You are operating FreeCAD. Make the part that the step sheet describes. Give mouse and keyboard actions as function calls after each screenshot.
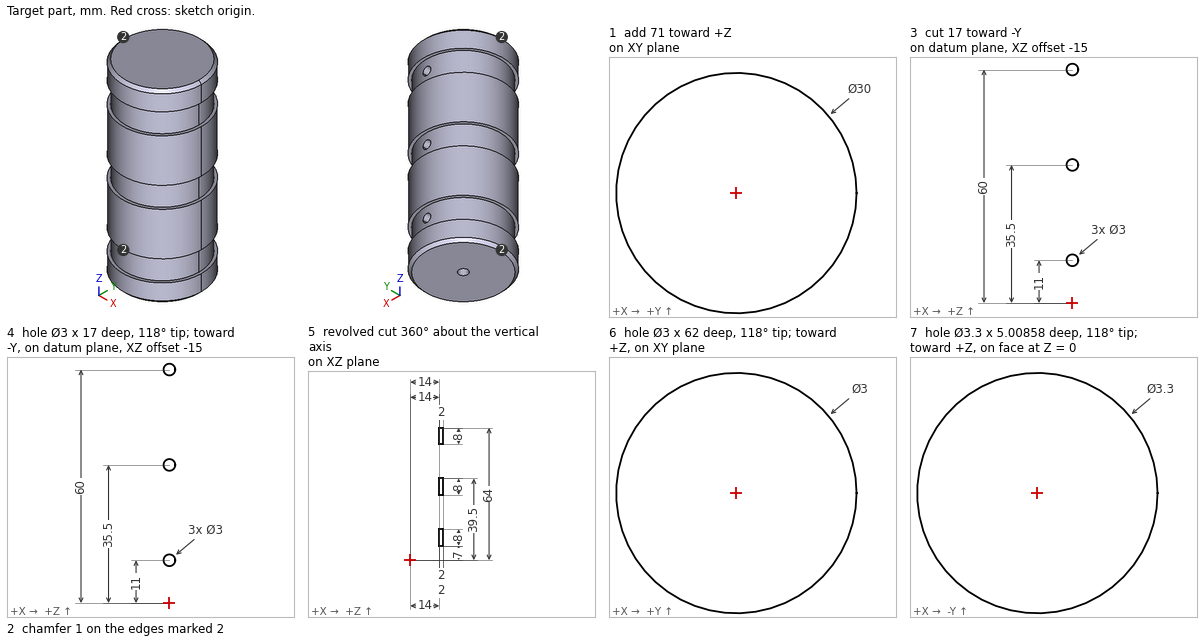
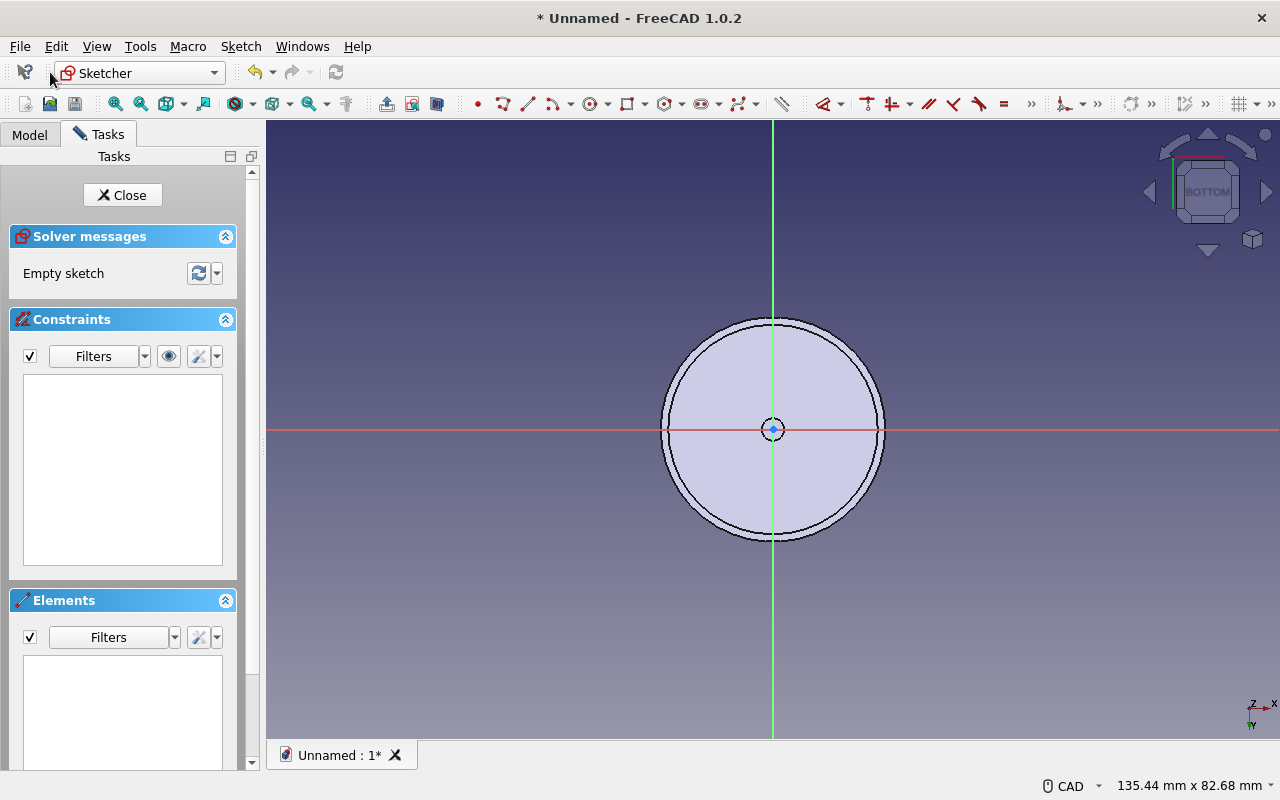
scroll(777, 430, up, 14)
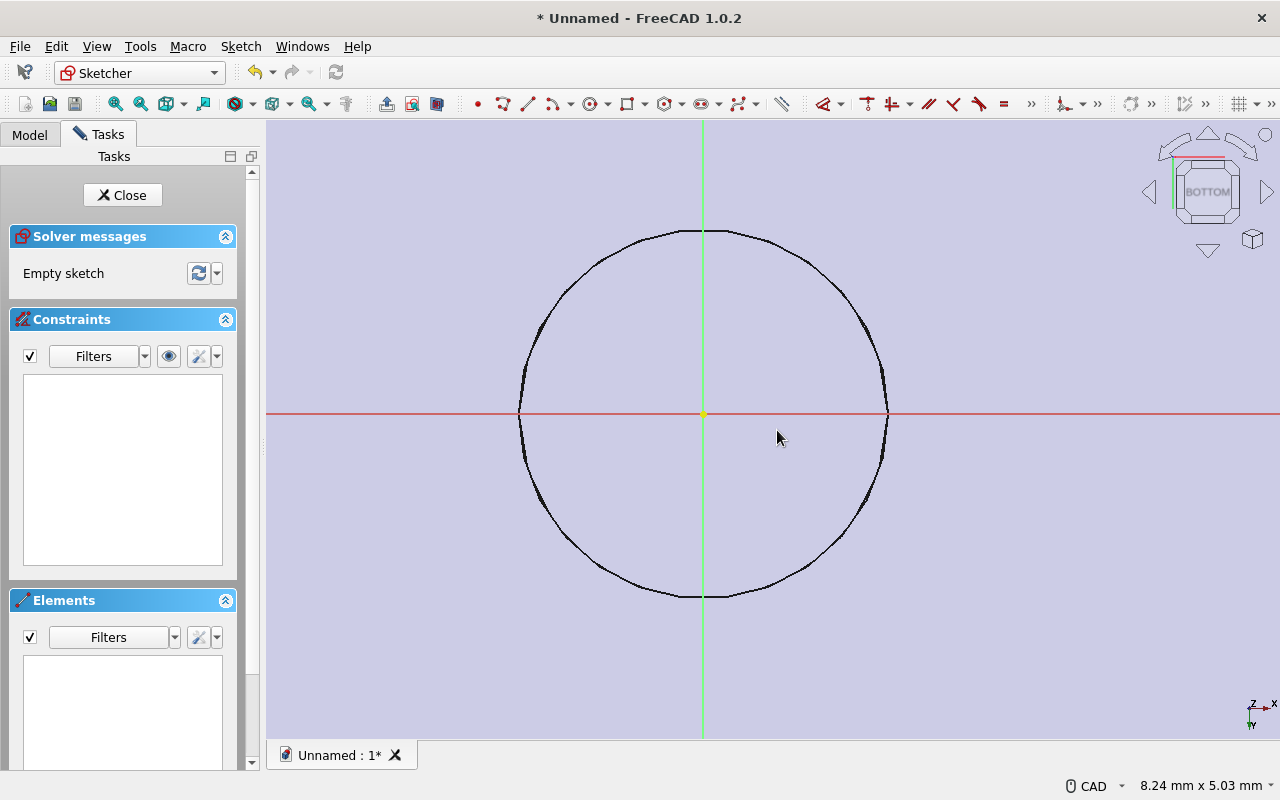
click(590, 104)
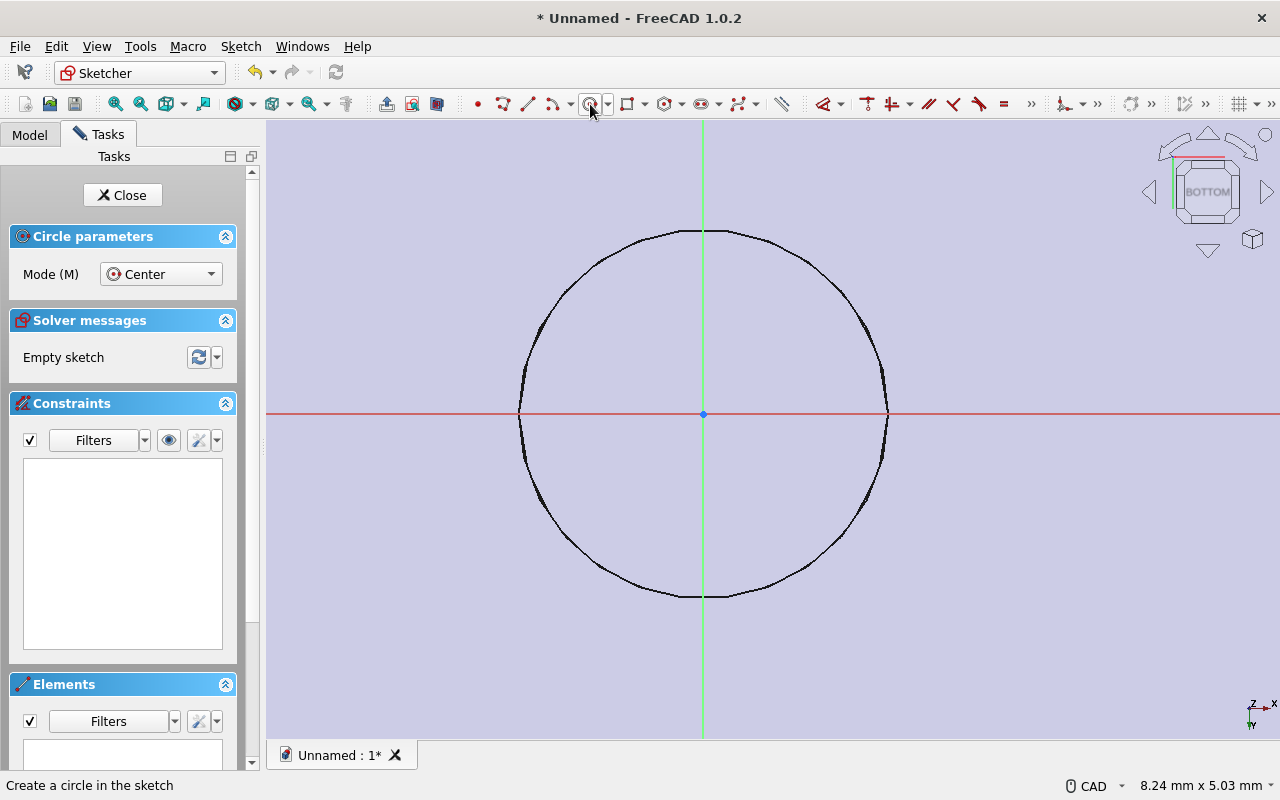
click(703, 414)
move(847, 270)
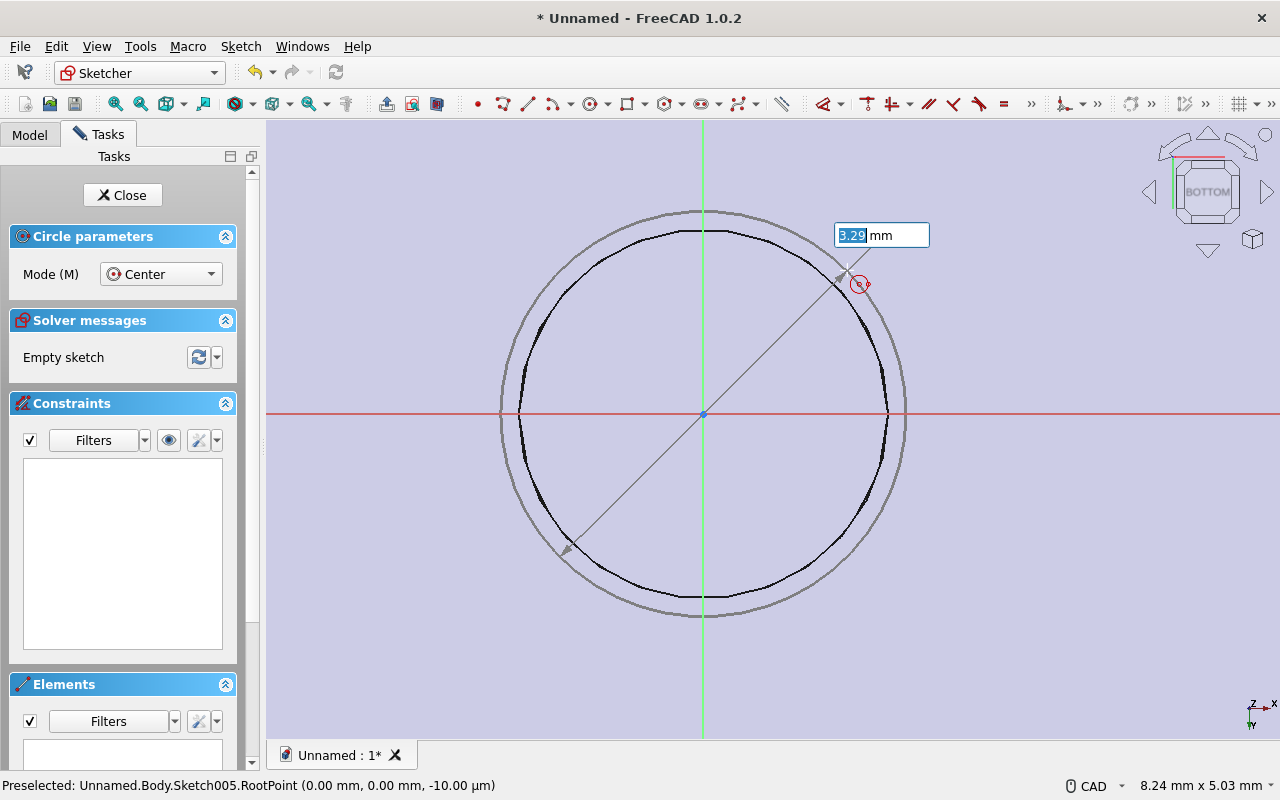
text(3.3)
key(Return)
key(Escape)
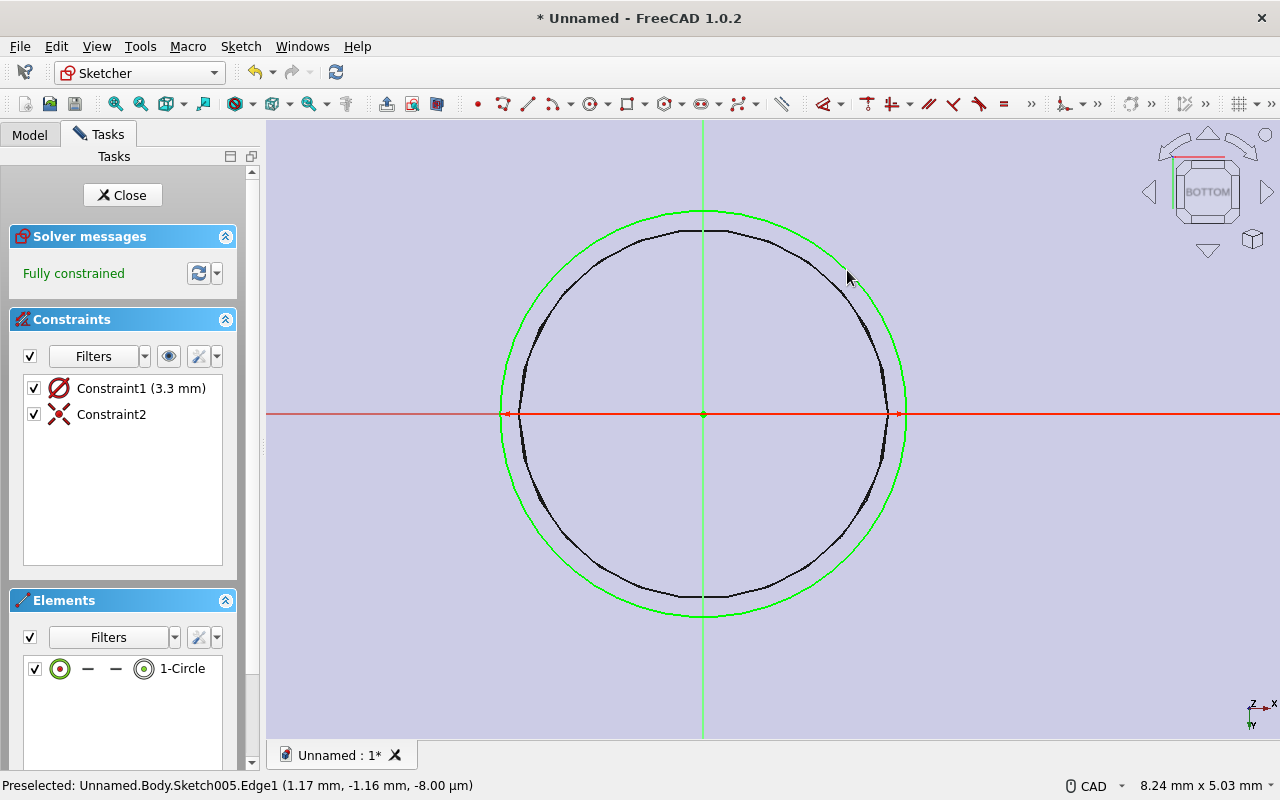
click(123, 195)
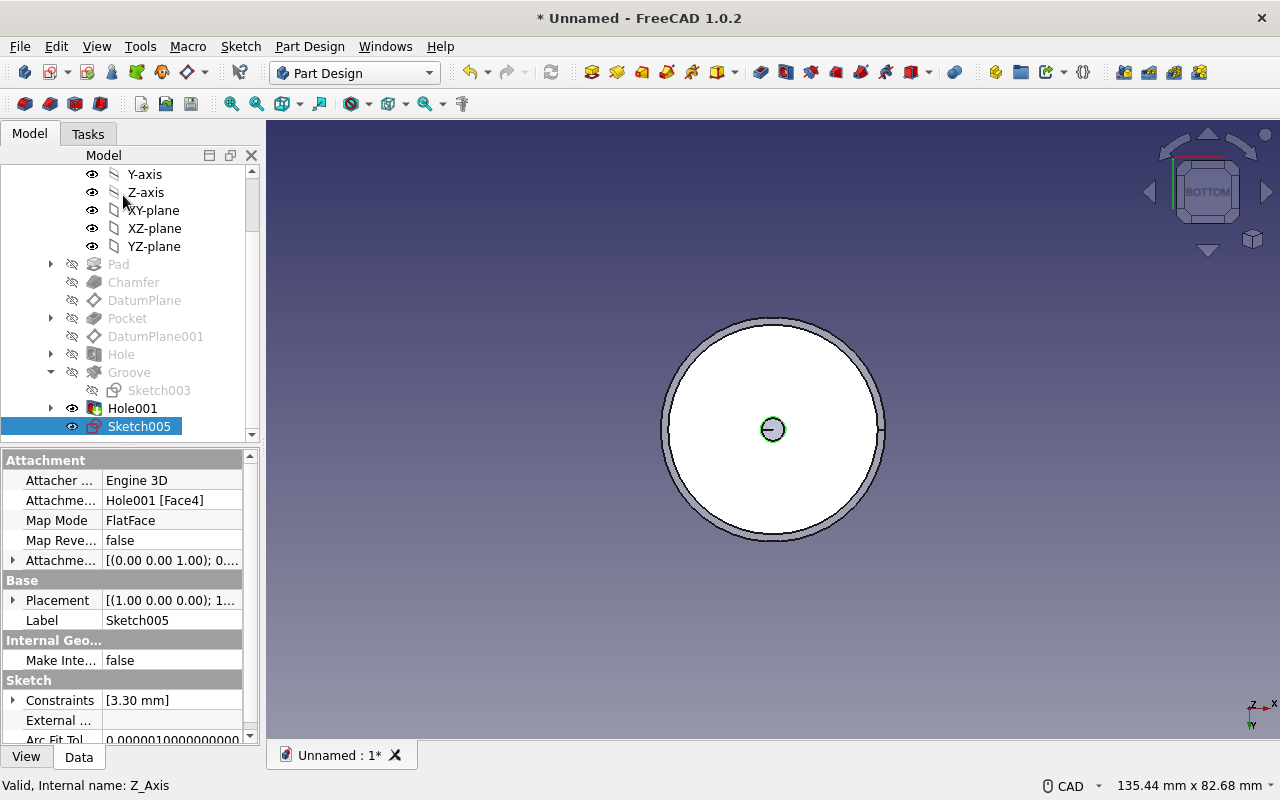
click(786, 72)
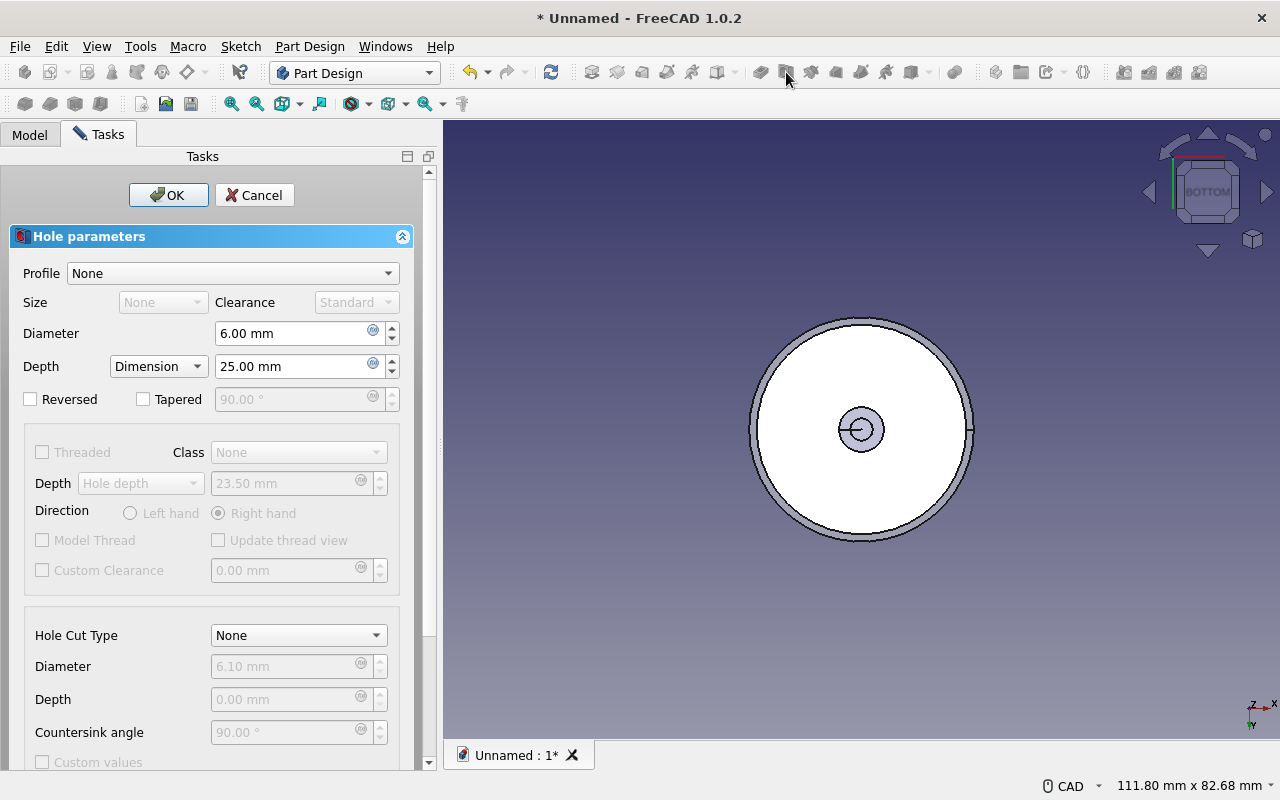
triple_click(300, 334)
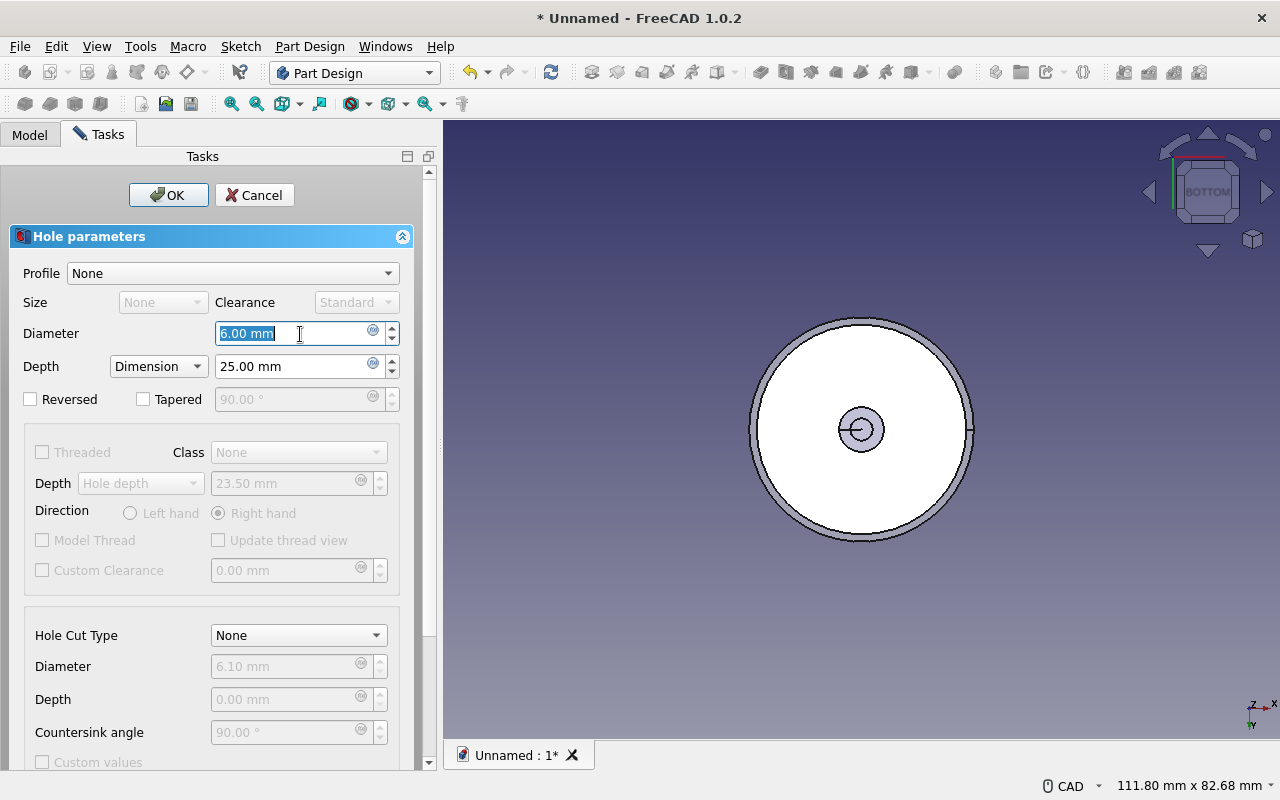
text(3.3)
key(Tab)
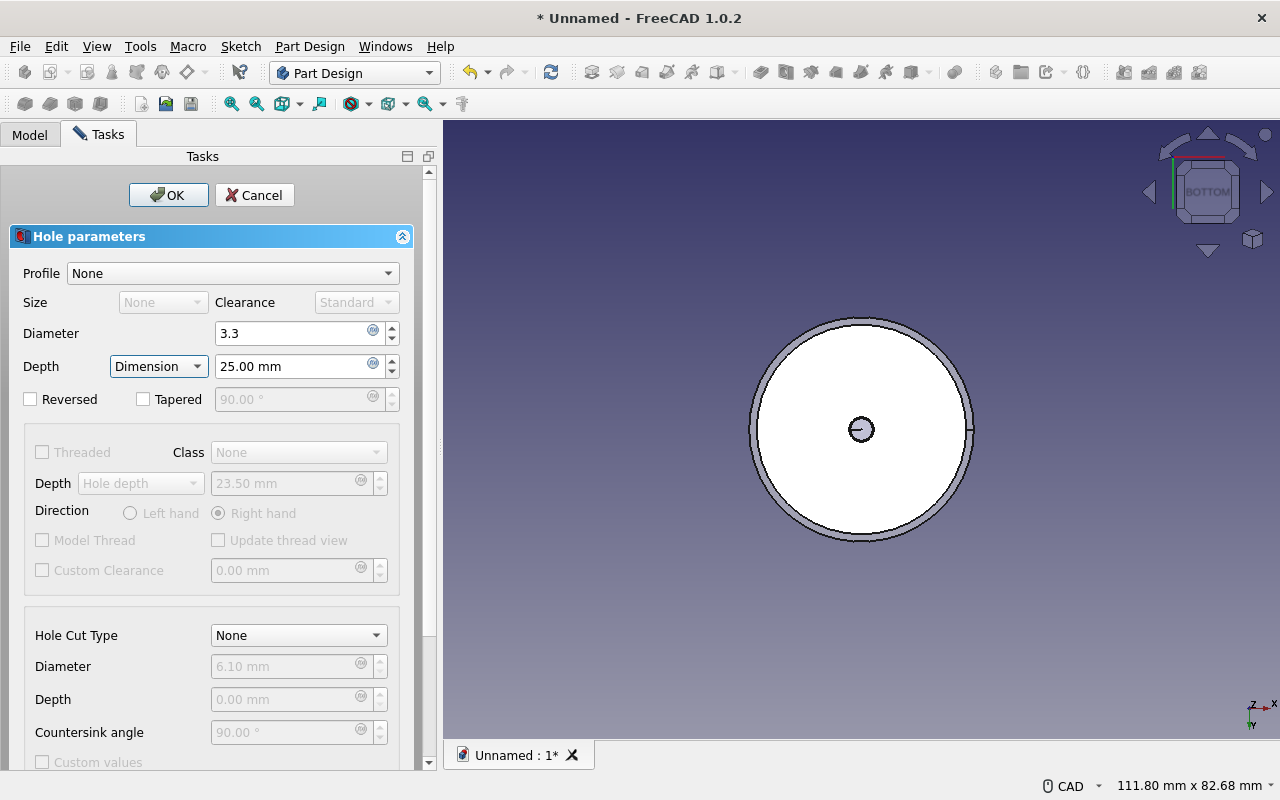
triple_click(300, 366)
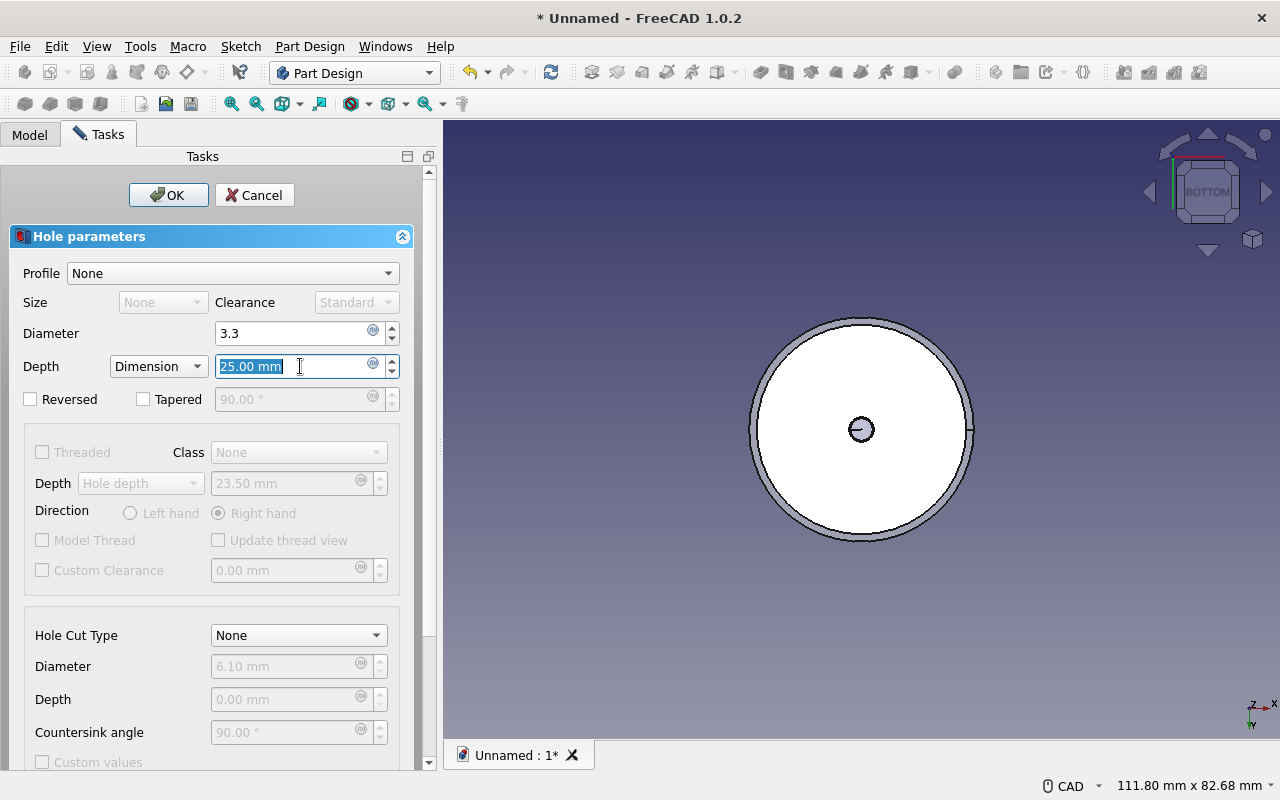
text(5.00858)
key(Tab)